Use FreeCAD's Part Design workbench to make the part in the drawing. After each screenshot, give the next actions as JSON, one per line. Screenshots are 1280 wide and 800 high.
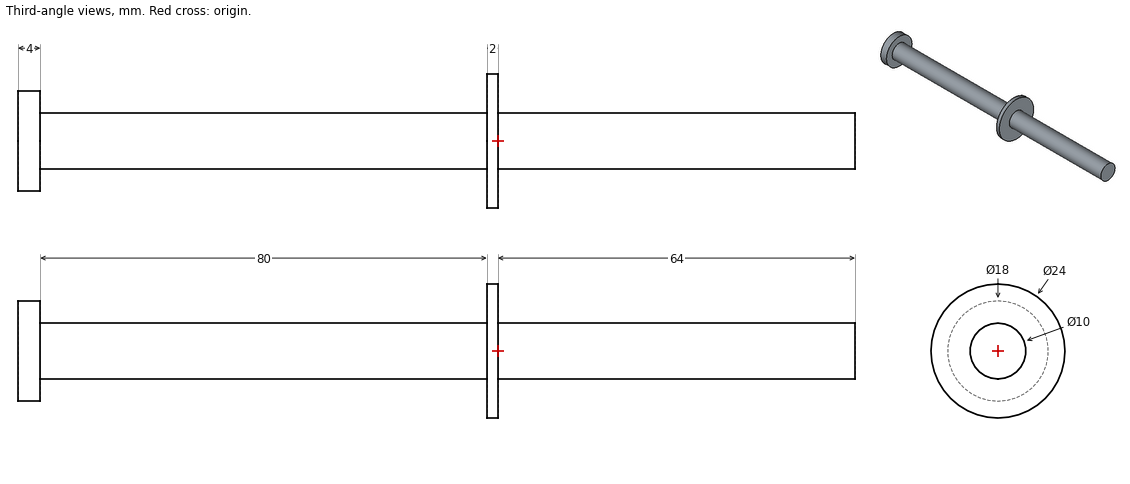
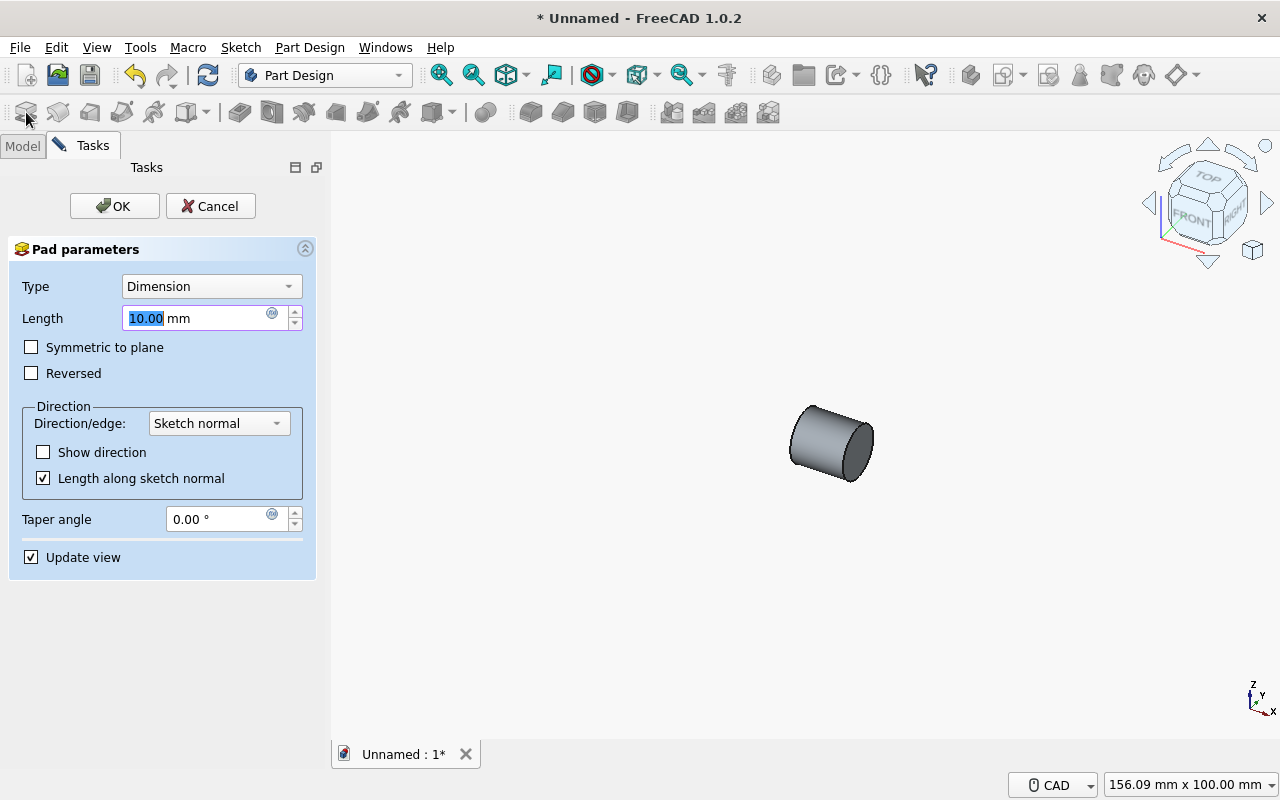
{"action": "type", "text": "64"}
{"action": "key", "text": "Tab"}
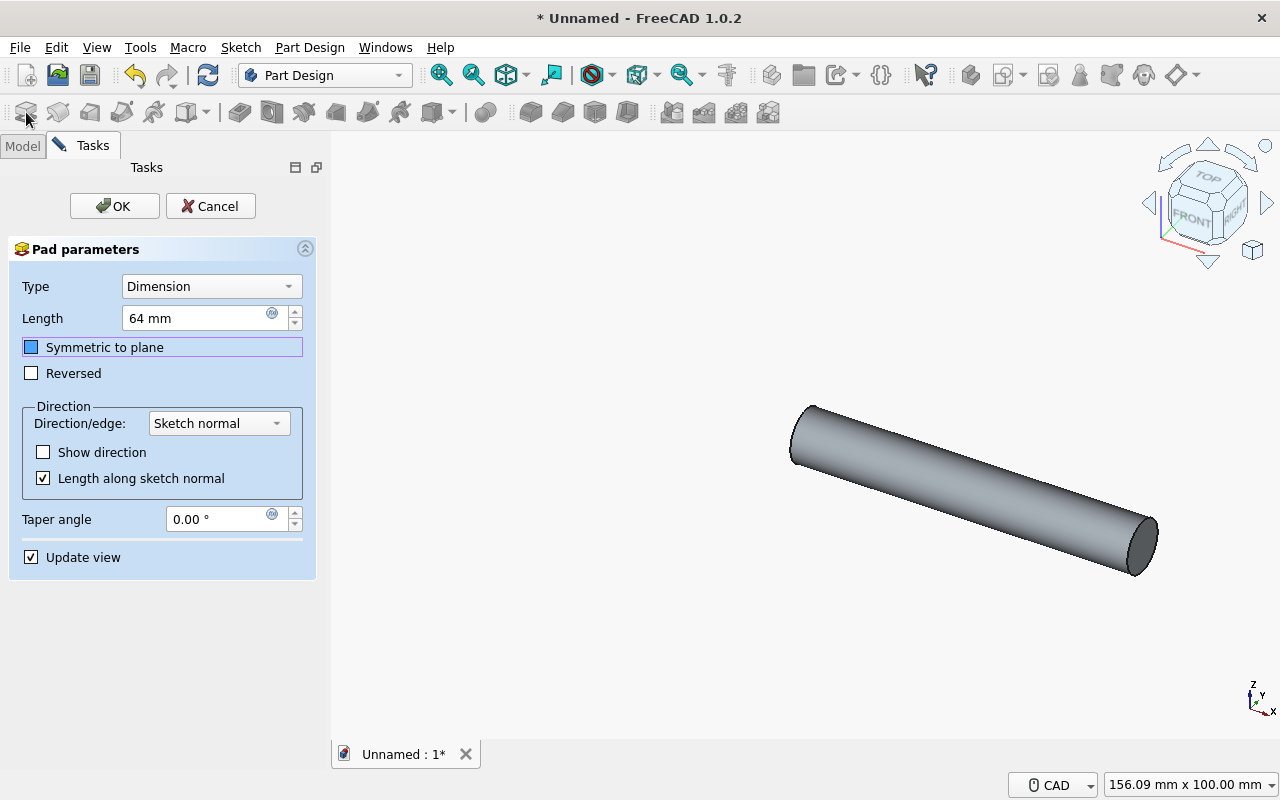
{"action": "left_click", "coordinate": [115, 206]}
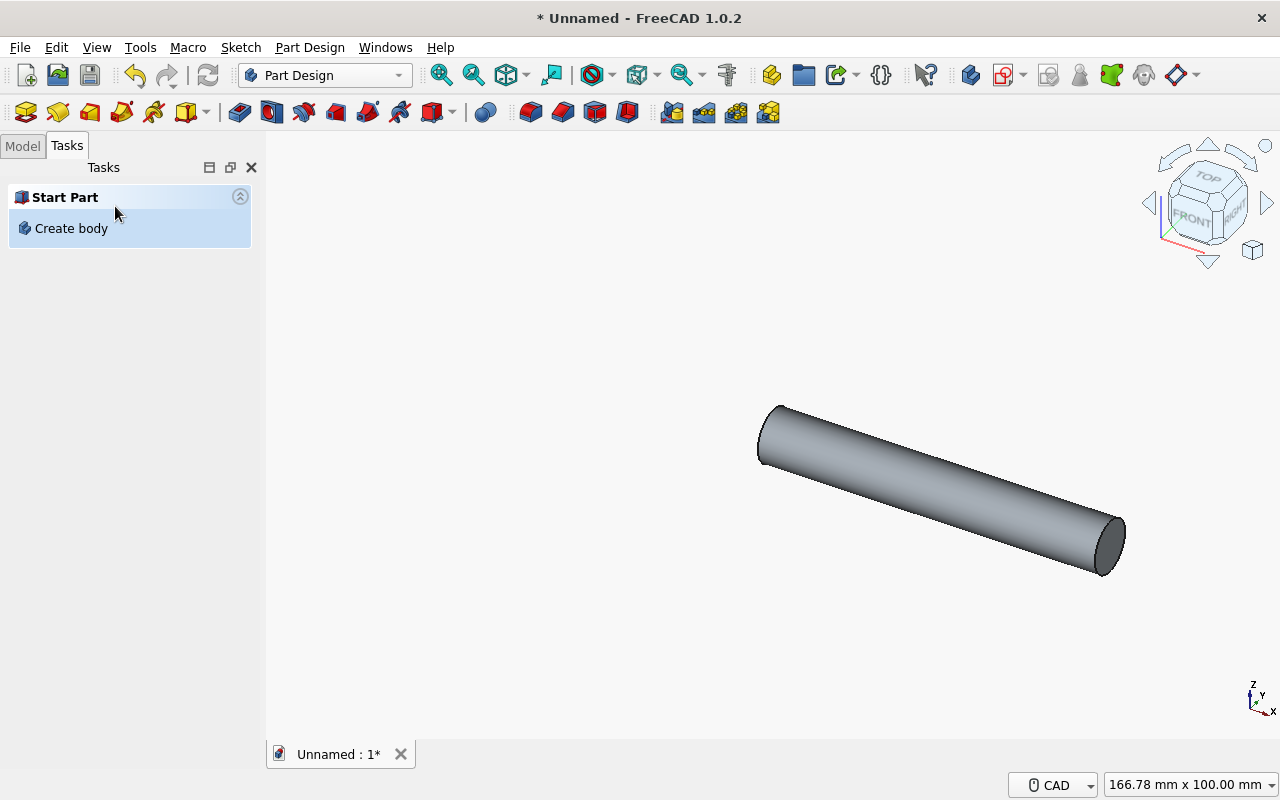
{"action": "key", "text": "v f"}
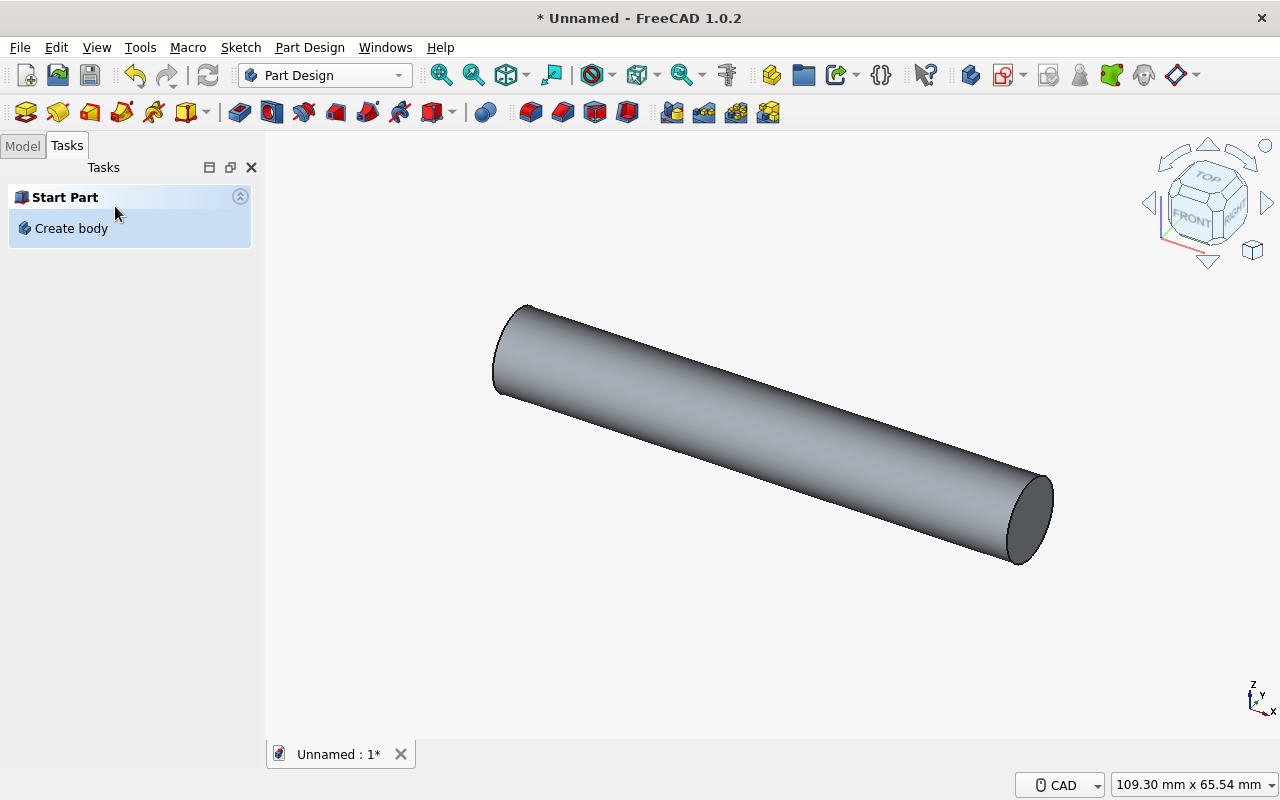
{"action": "left_click", "coordinate": [1004, 76]}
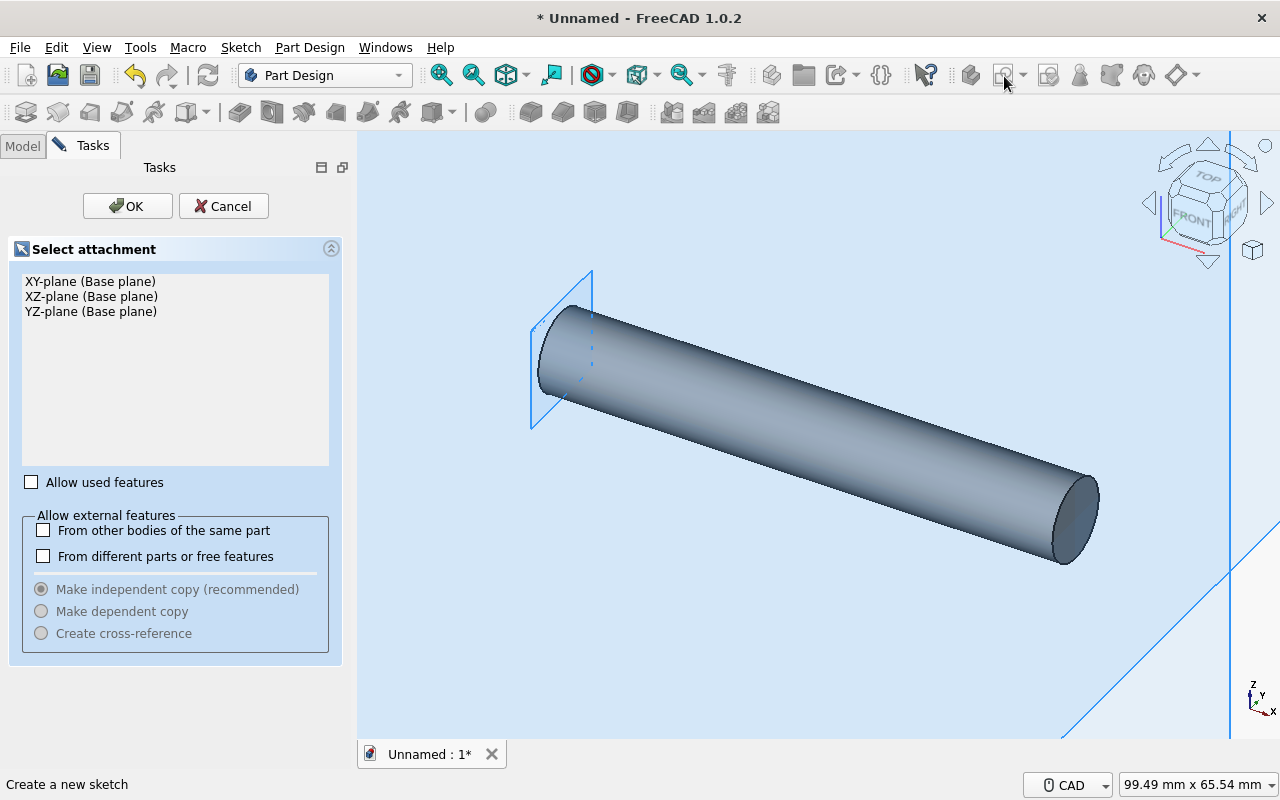
{"action": "left_click", "coordinate": [82, 312]}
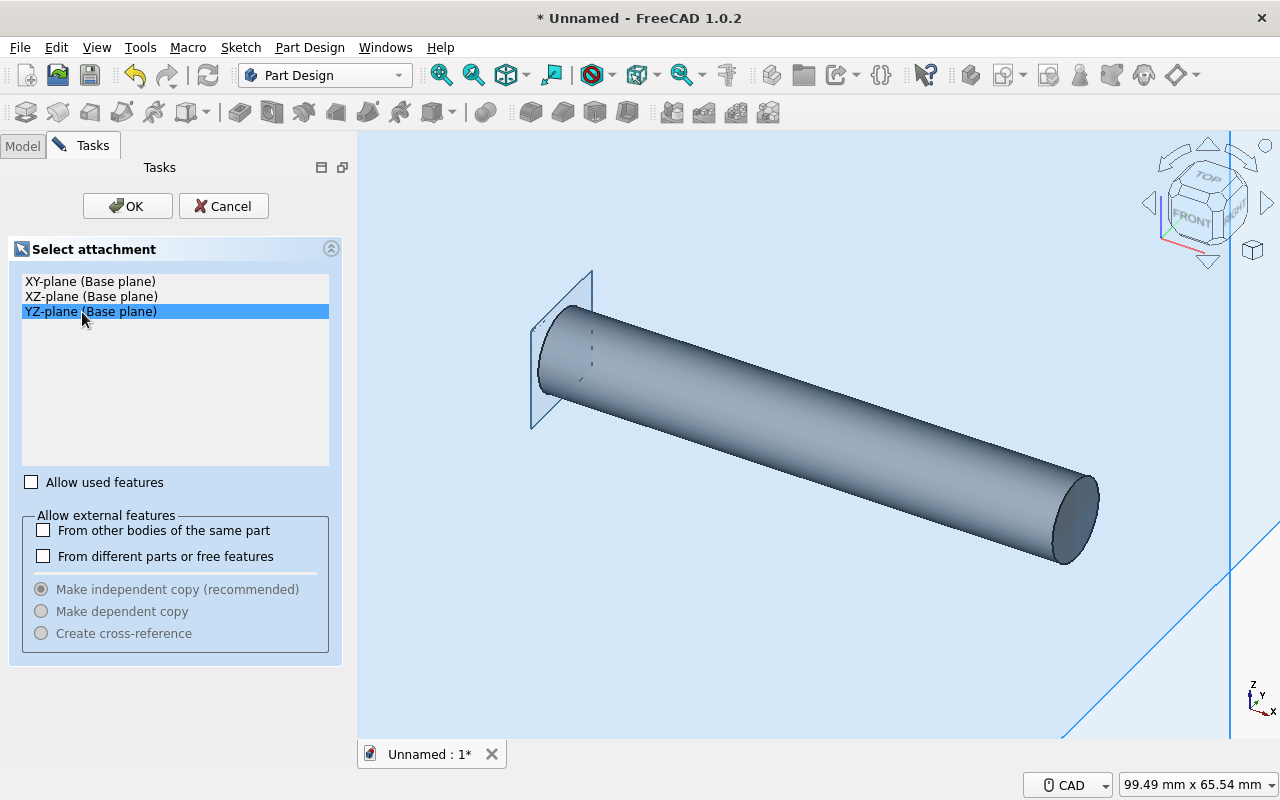
{"action": "left_click", "coordinate": [128, 206]}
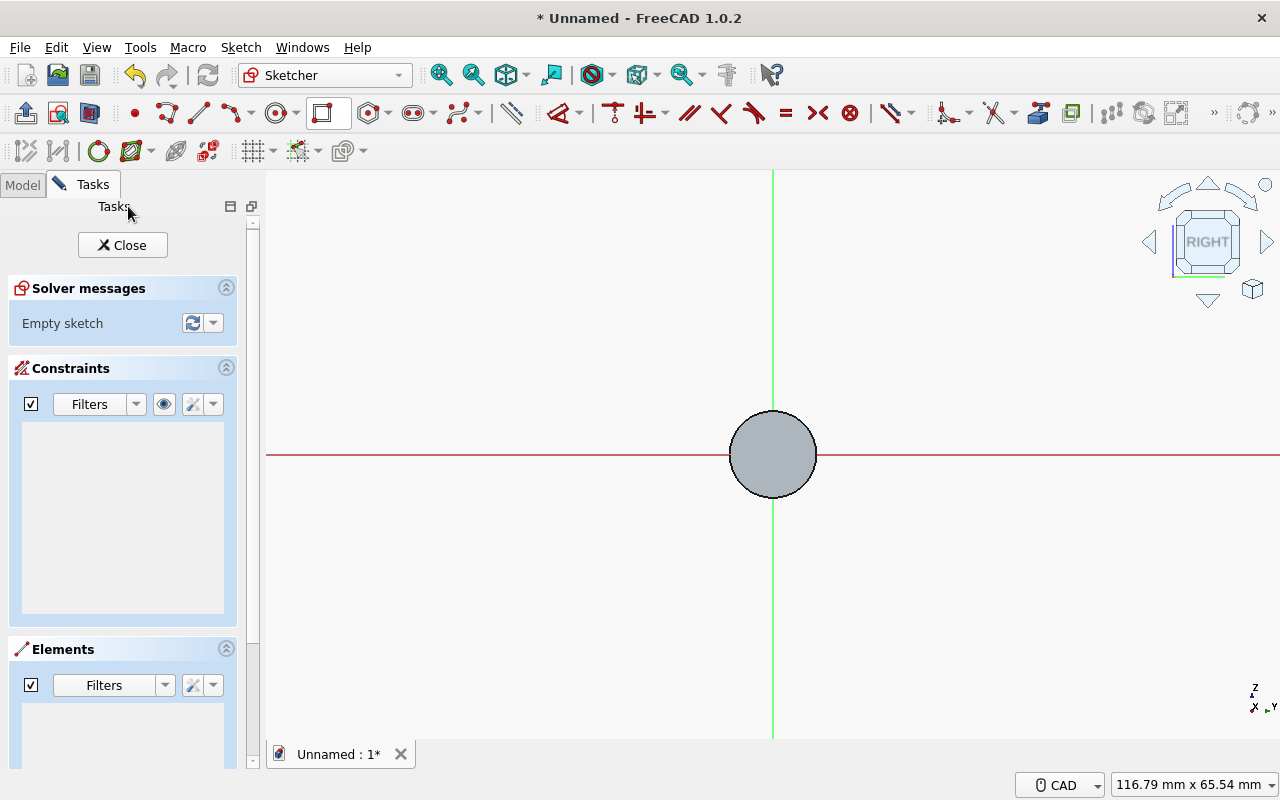
{"action": "key", "text": "q s"}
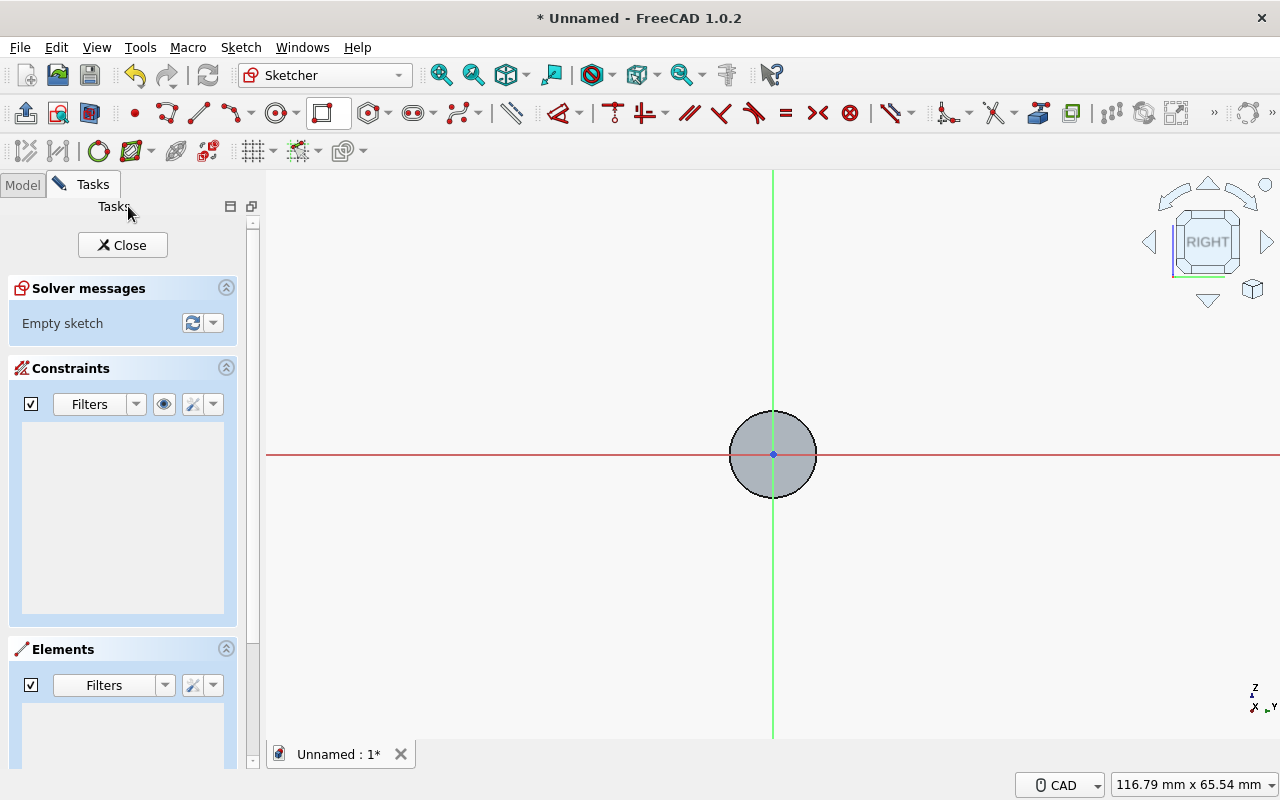
{"action": "scroll", "coordinate": [856, 454], "scroll_direction": "up", "scroll_amount": 3}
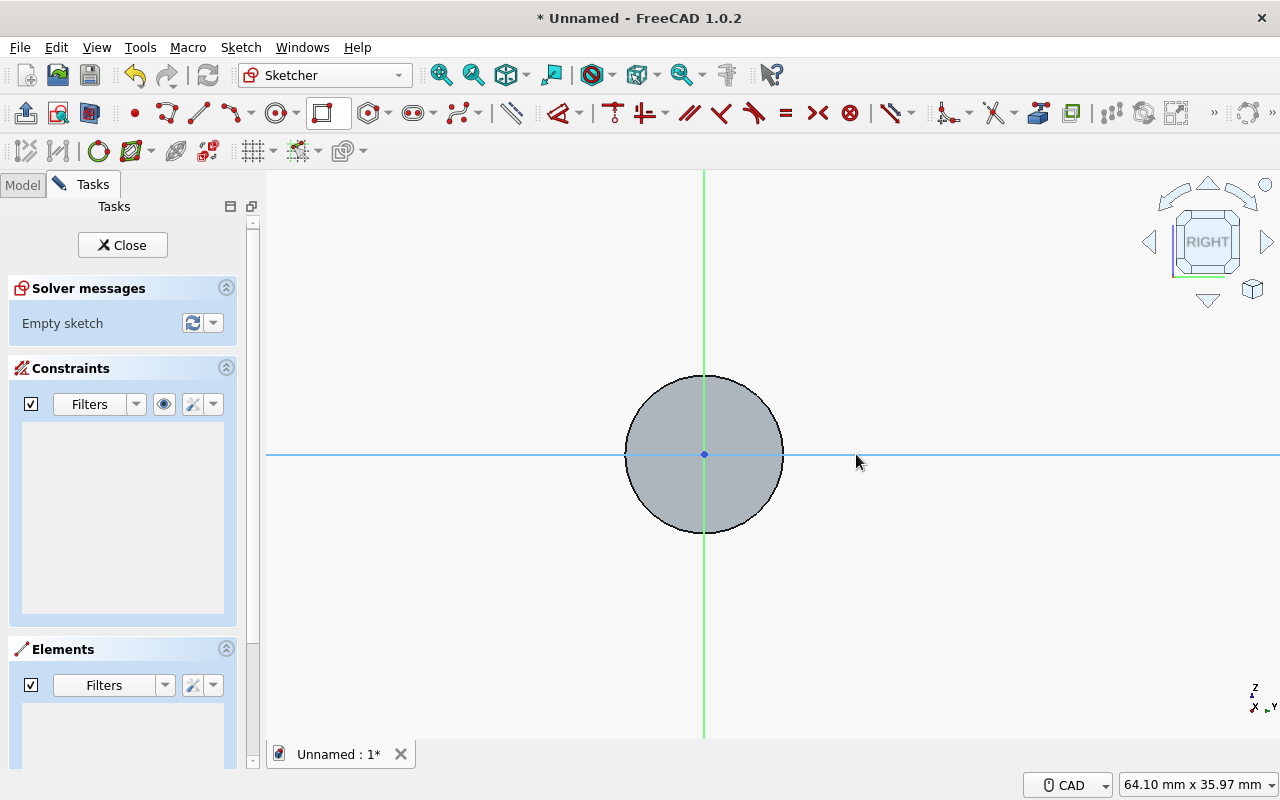
{"action": "left_click", "coordinate": [276, 114]}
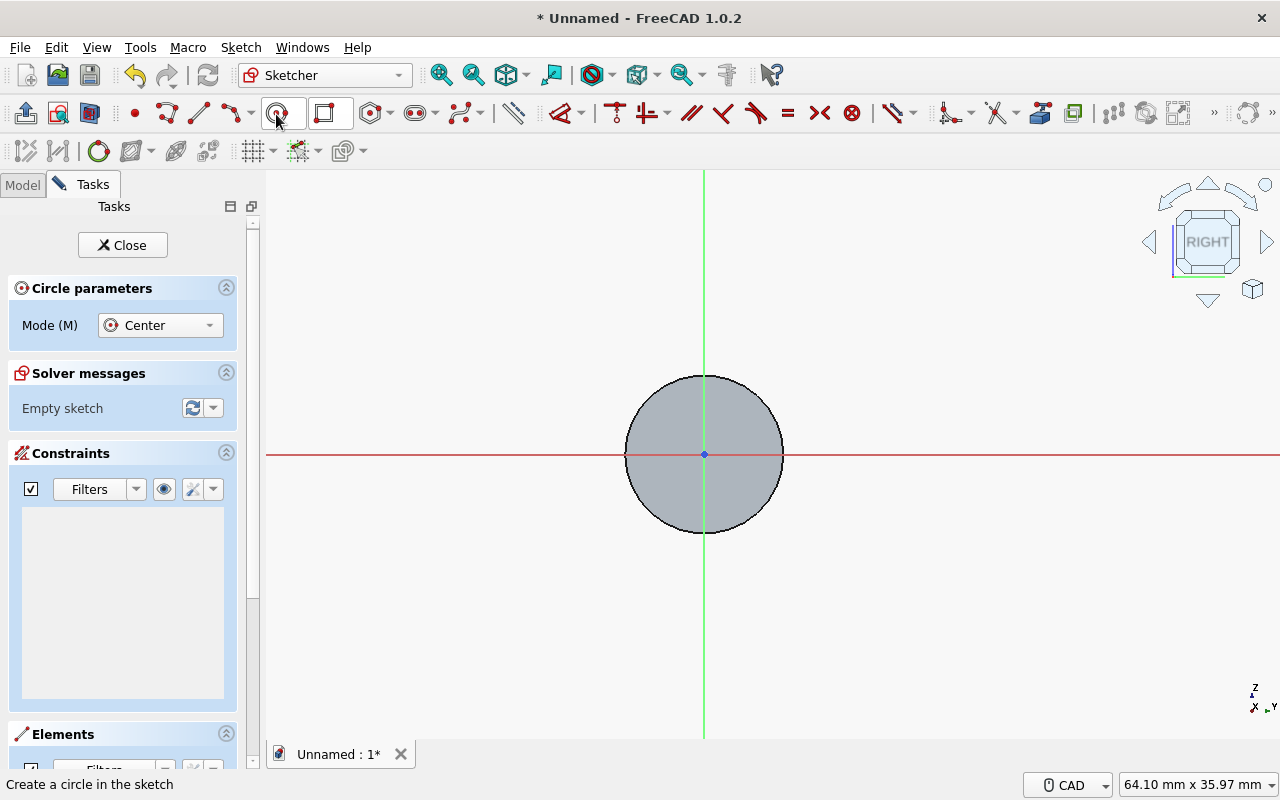
{"action": "left_click", "coordinate": [704, 454]}
{"action": "mouse_move", "coordinate": [839, 320]}